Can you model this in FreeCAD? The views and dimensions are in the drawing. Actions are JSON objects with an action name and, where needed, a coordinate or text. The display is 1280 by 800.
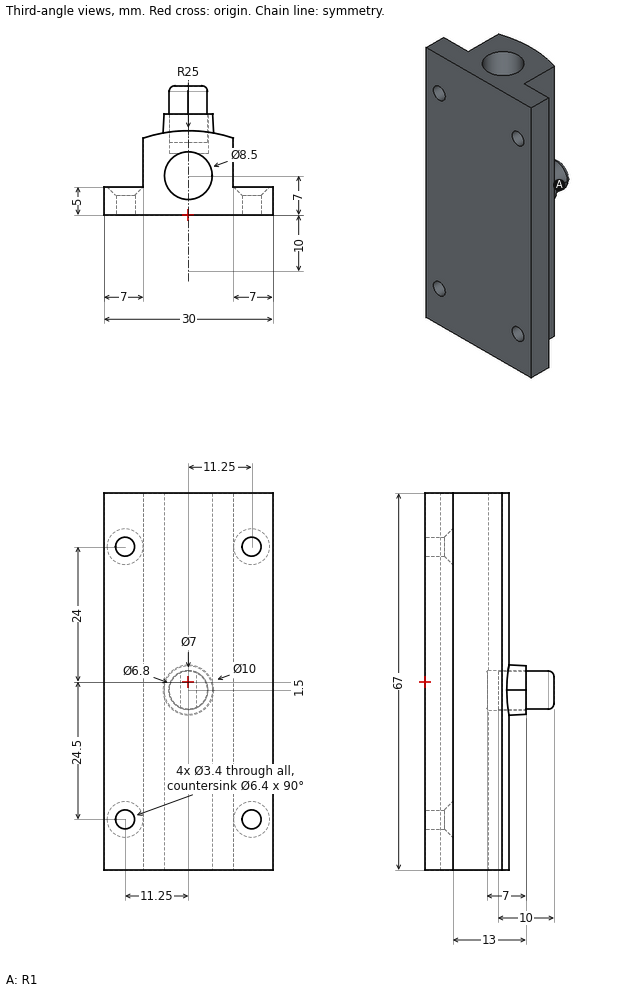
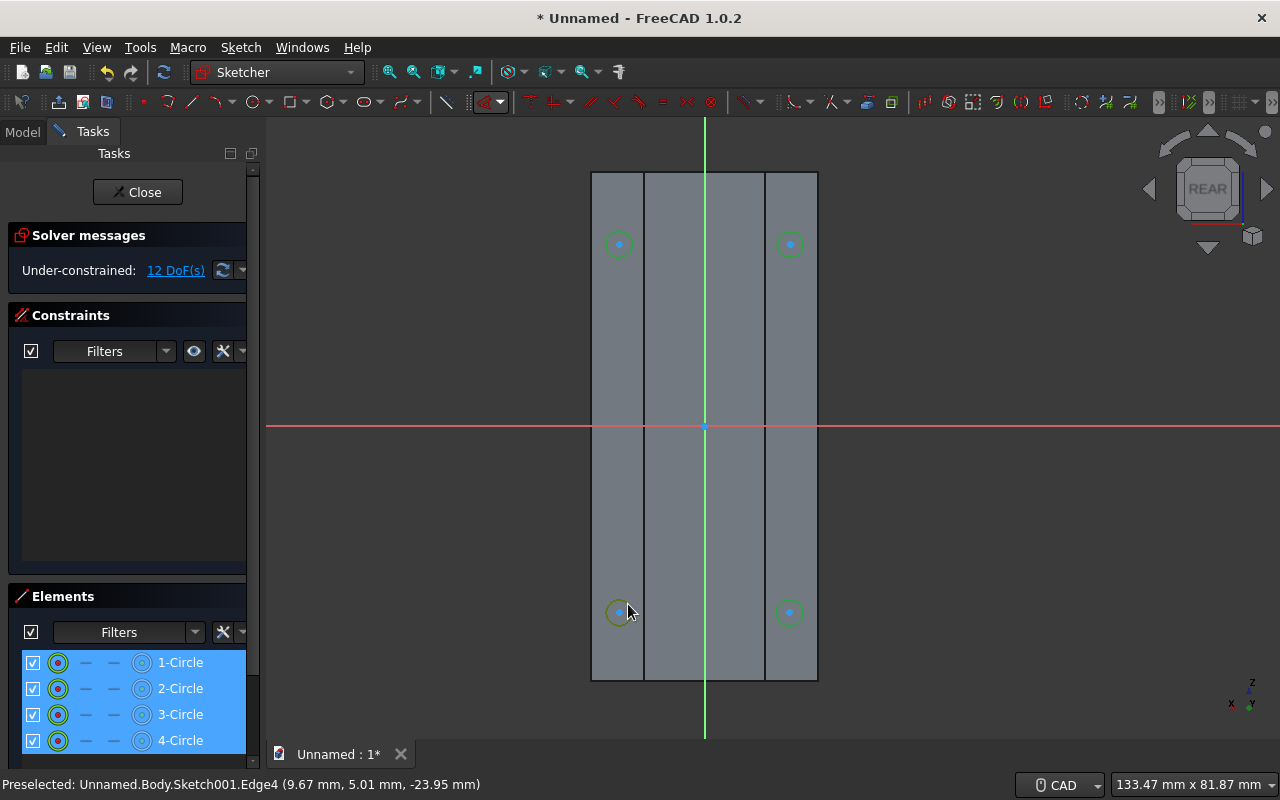
{"action": "left_click", "coordinate": [664, 102]}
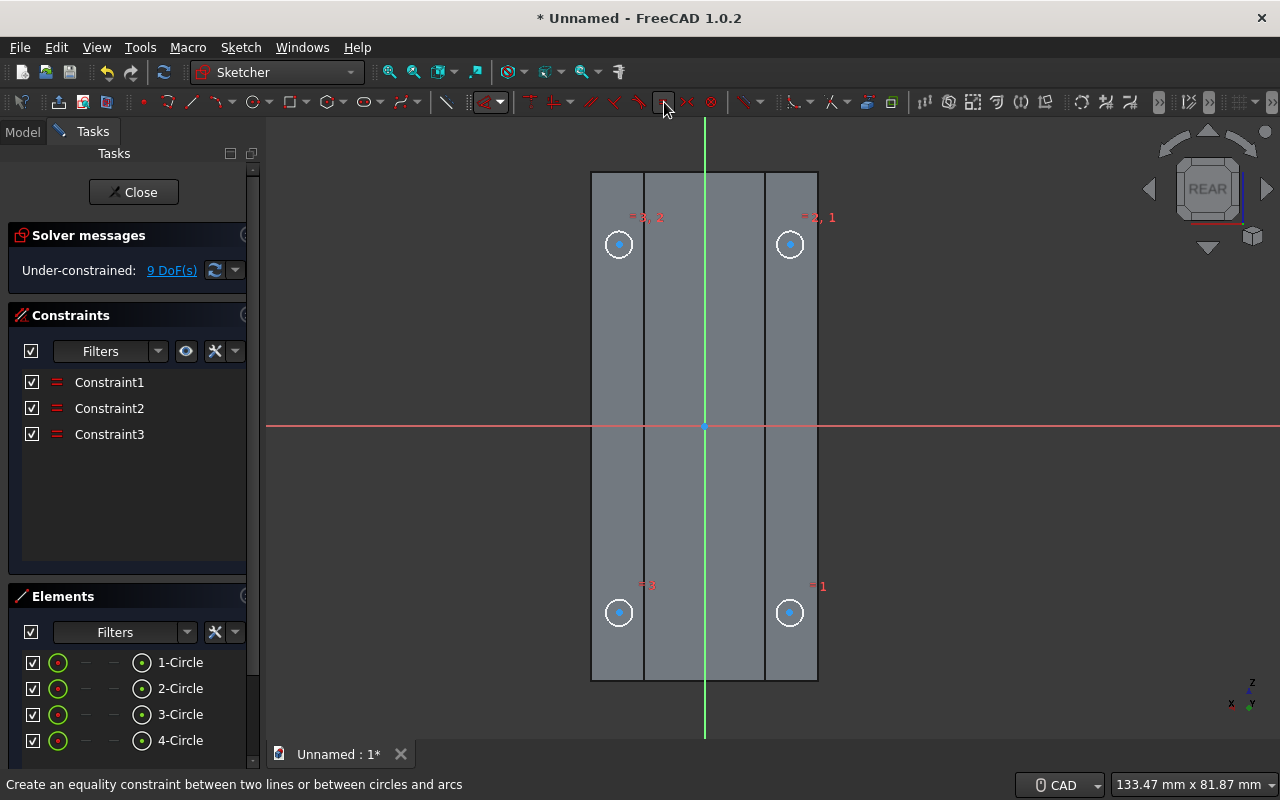
{"action": "left_click", "coordinate": [790, 613]}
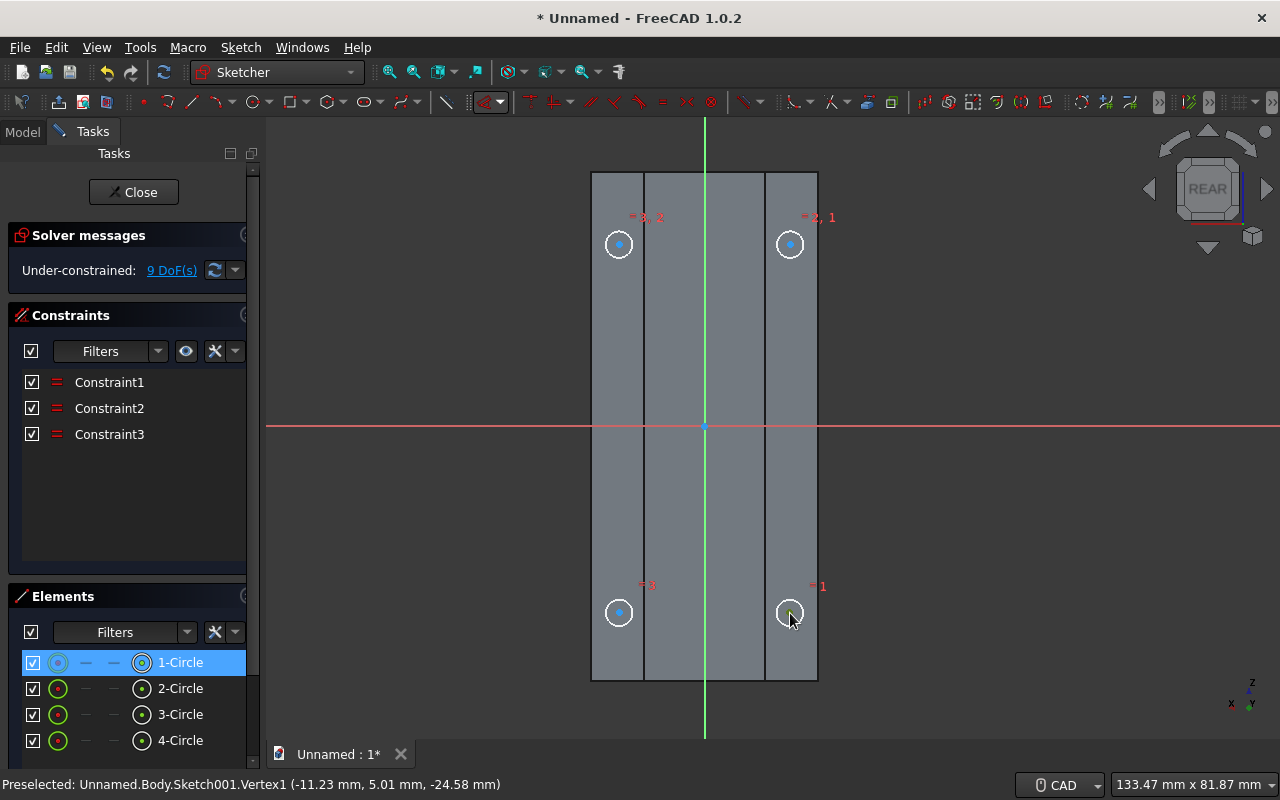
{"action": "left_click", "coordinate": [790, 245]}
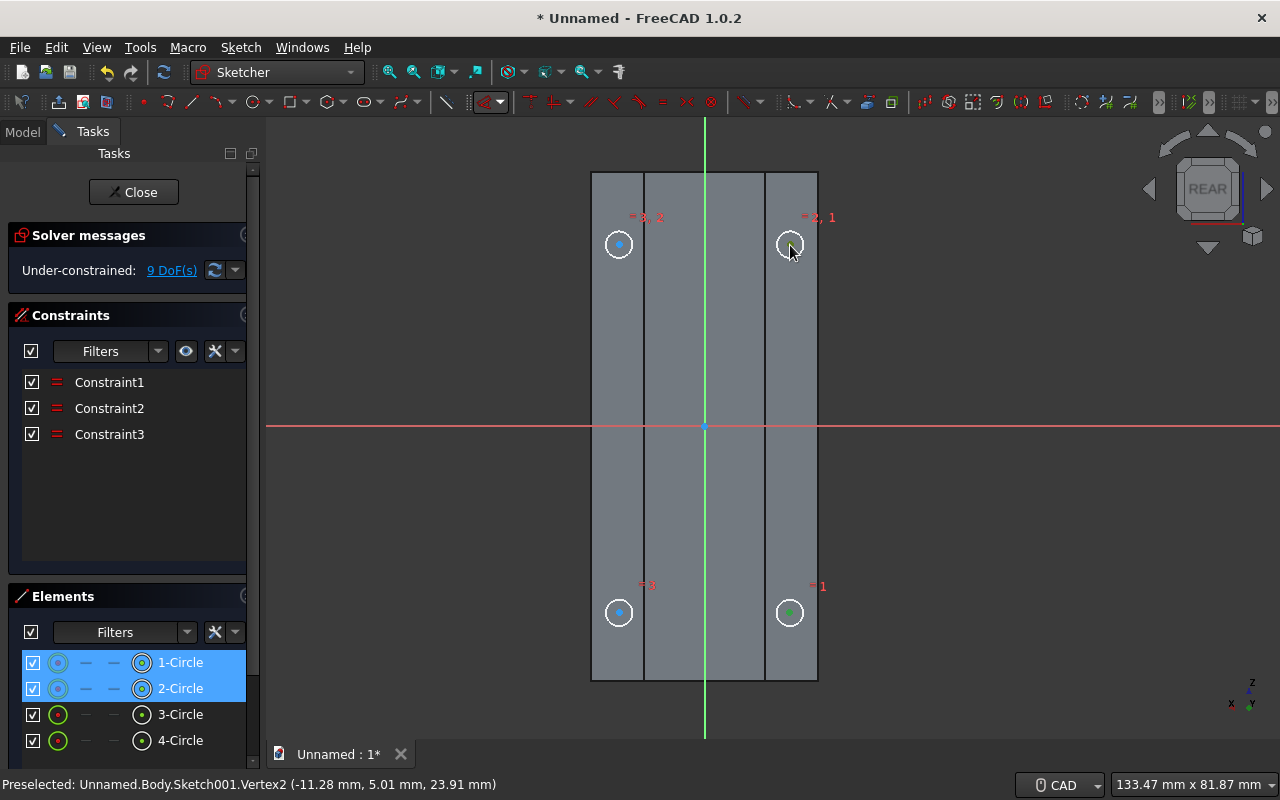
{"action": "key", "text": "v"}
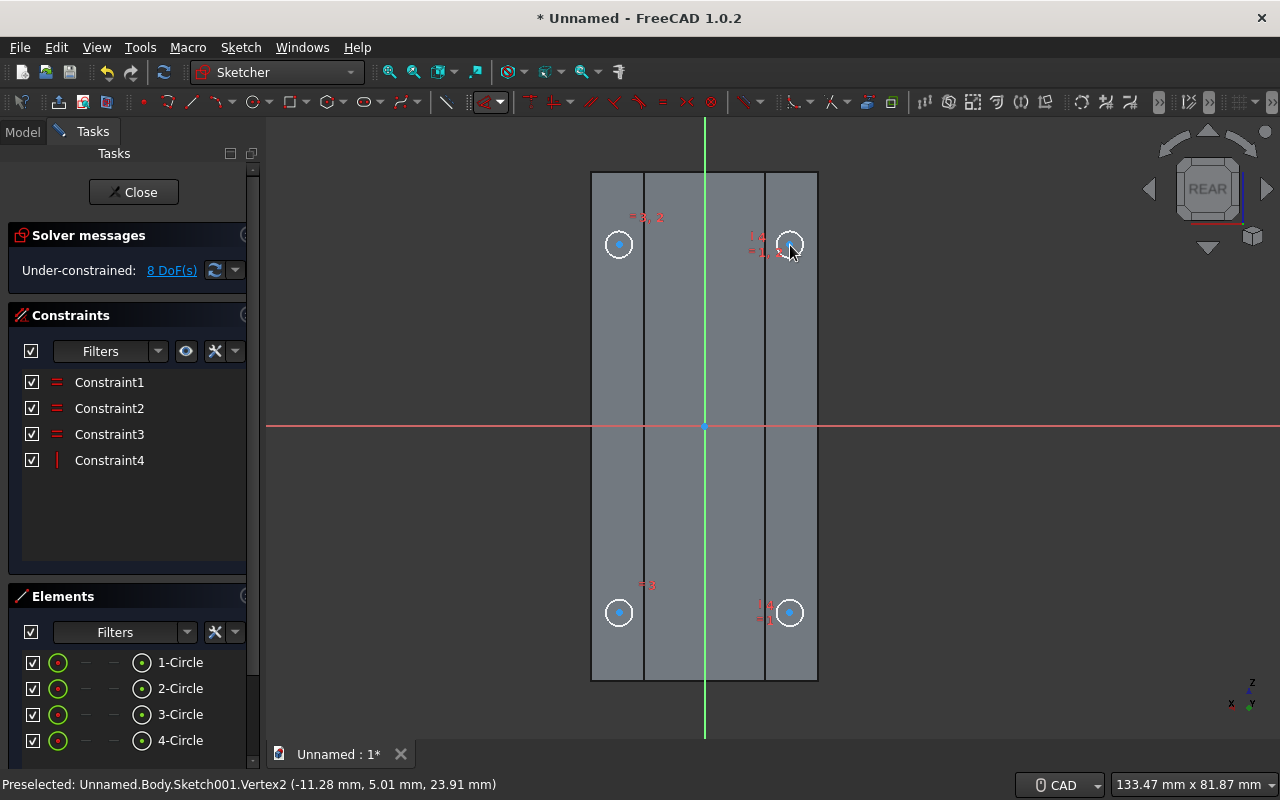
{"action": "left_click", "coordinate": [790, 245]}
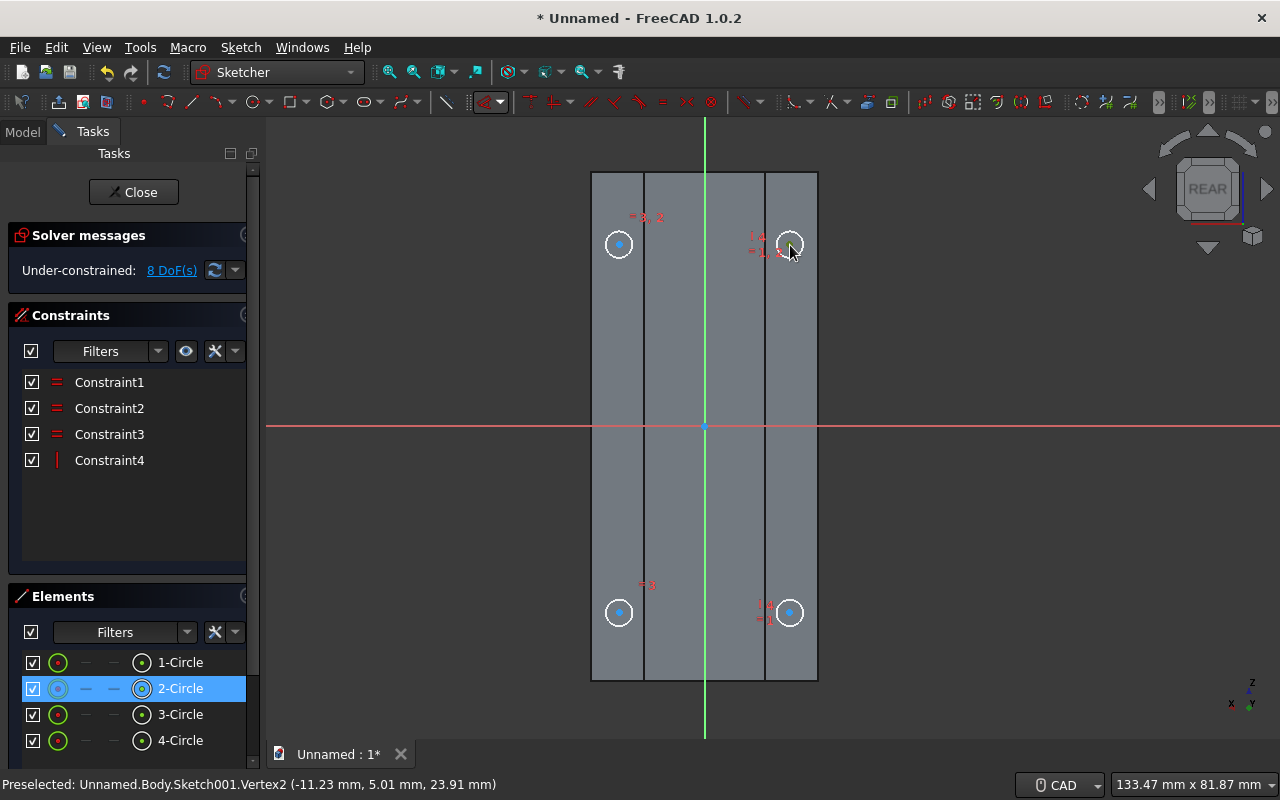
{"action": "left_click", "coordinate": [619, 245]}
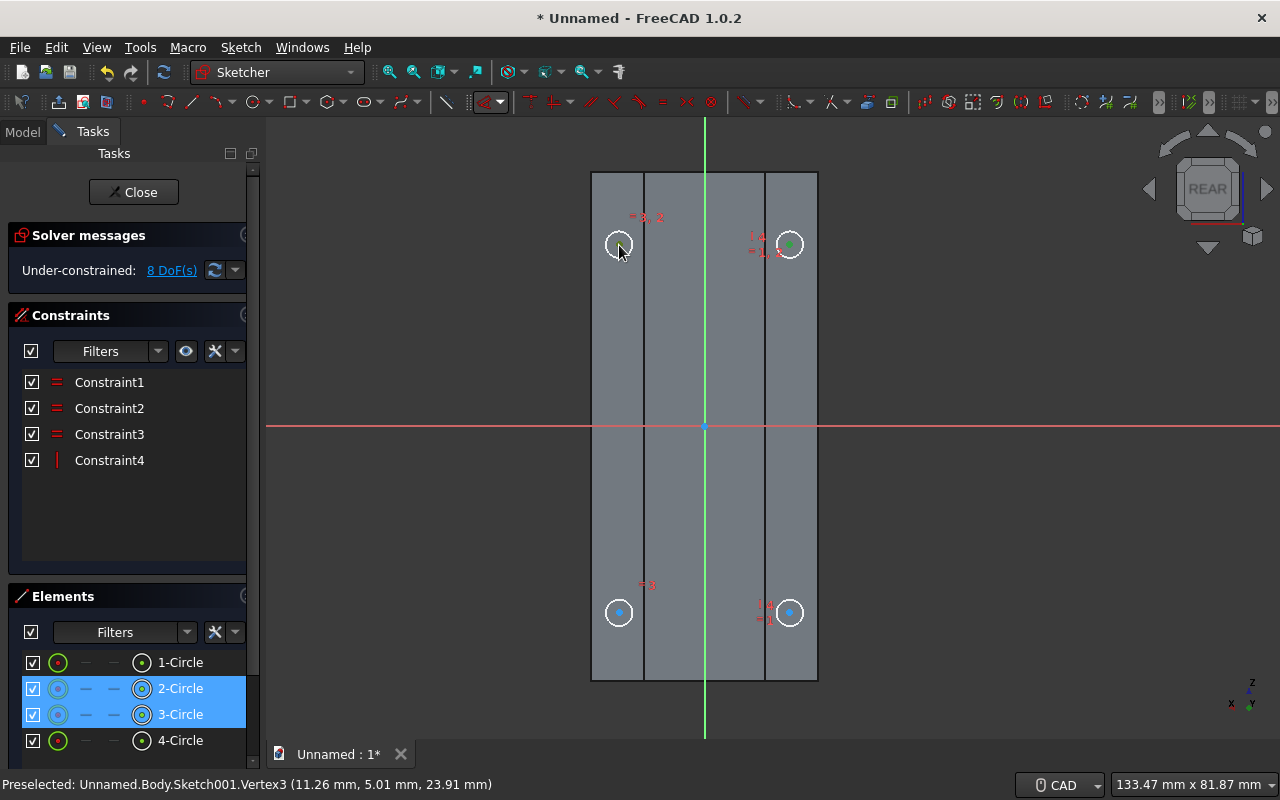
{"action": "key", "text": "h"}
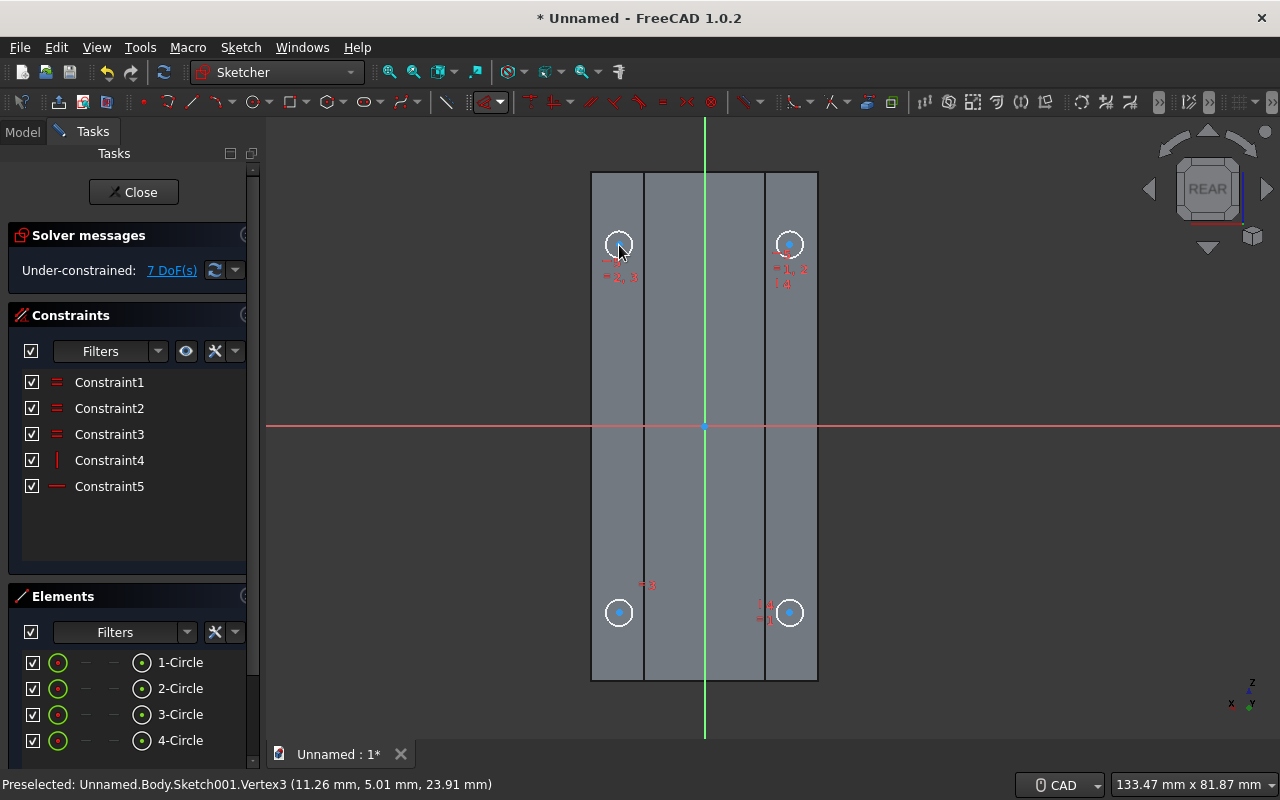
{"action": "left_click", "coordinate": [619, 245]}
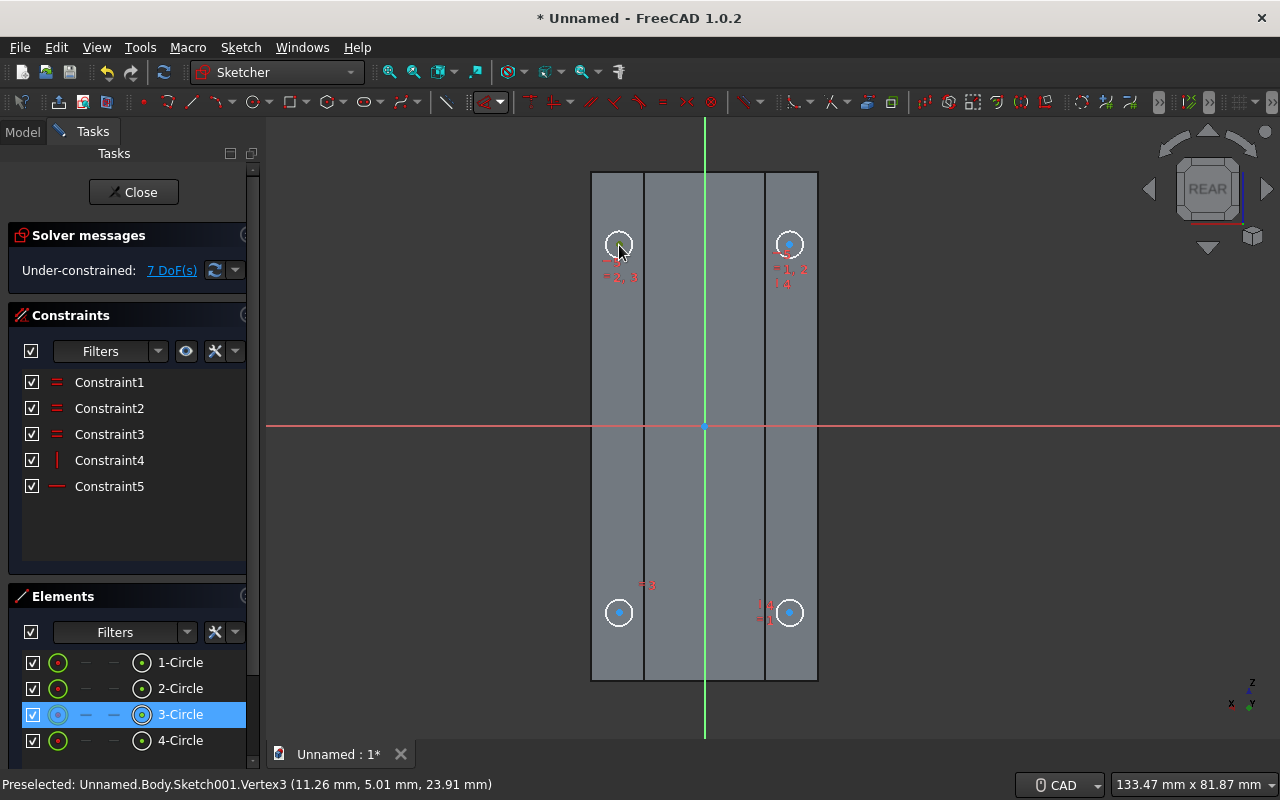
{"action": "left_click", "coordinate": [619, 613]}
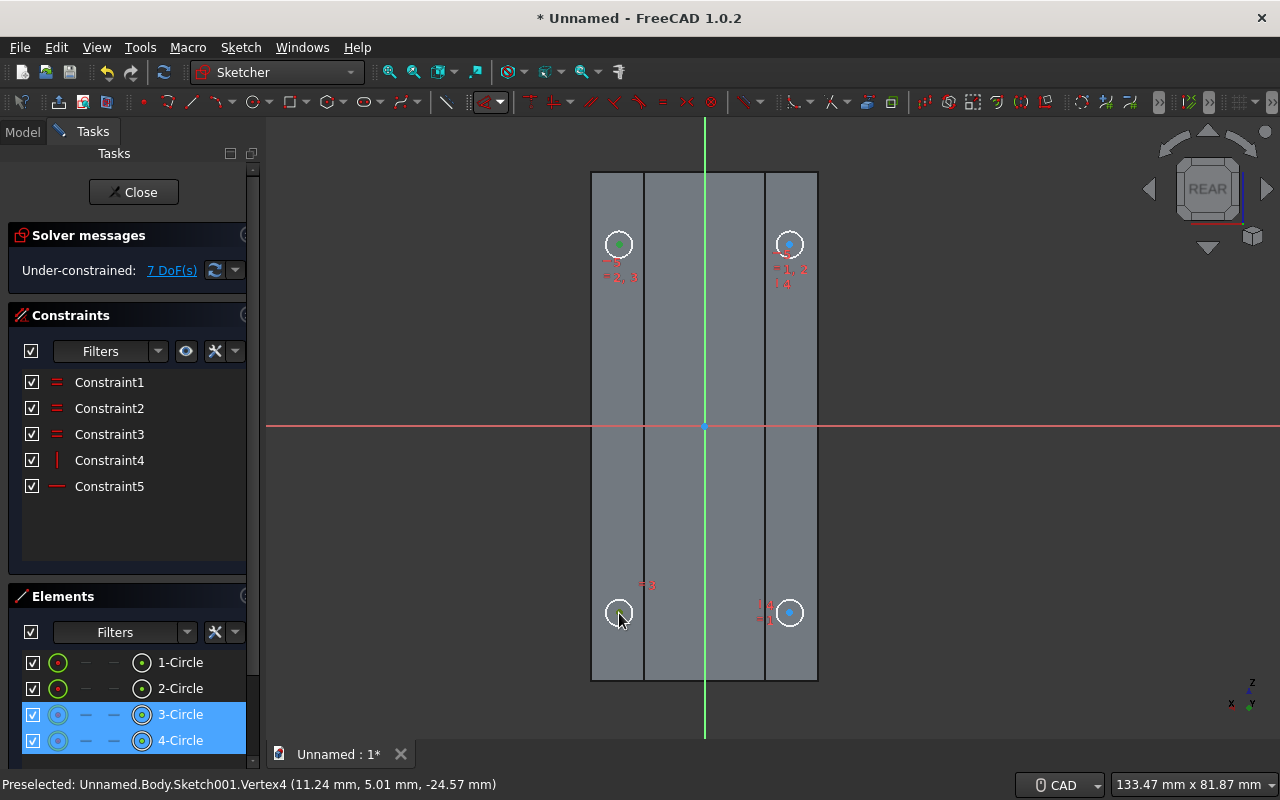
{"action": "key", "text": "v"}